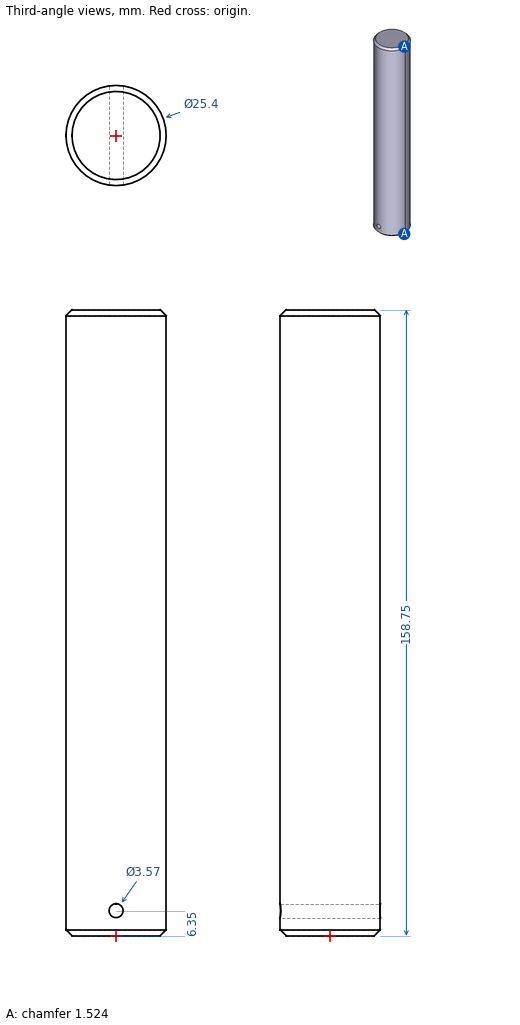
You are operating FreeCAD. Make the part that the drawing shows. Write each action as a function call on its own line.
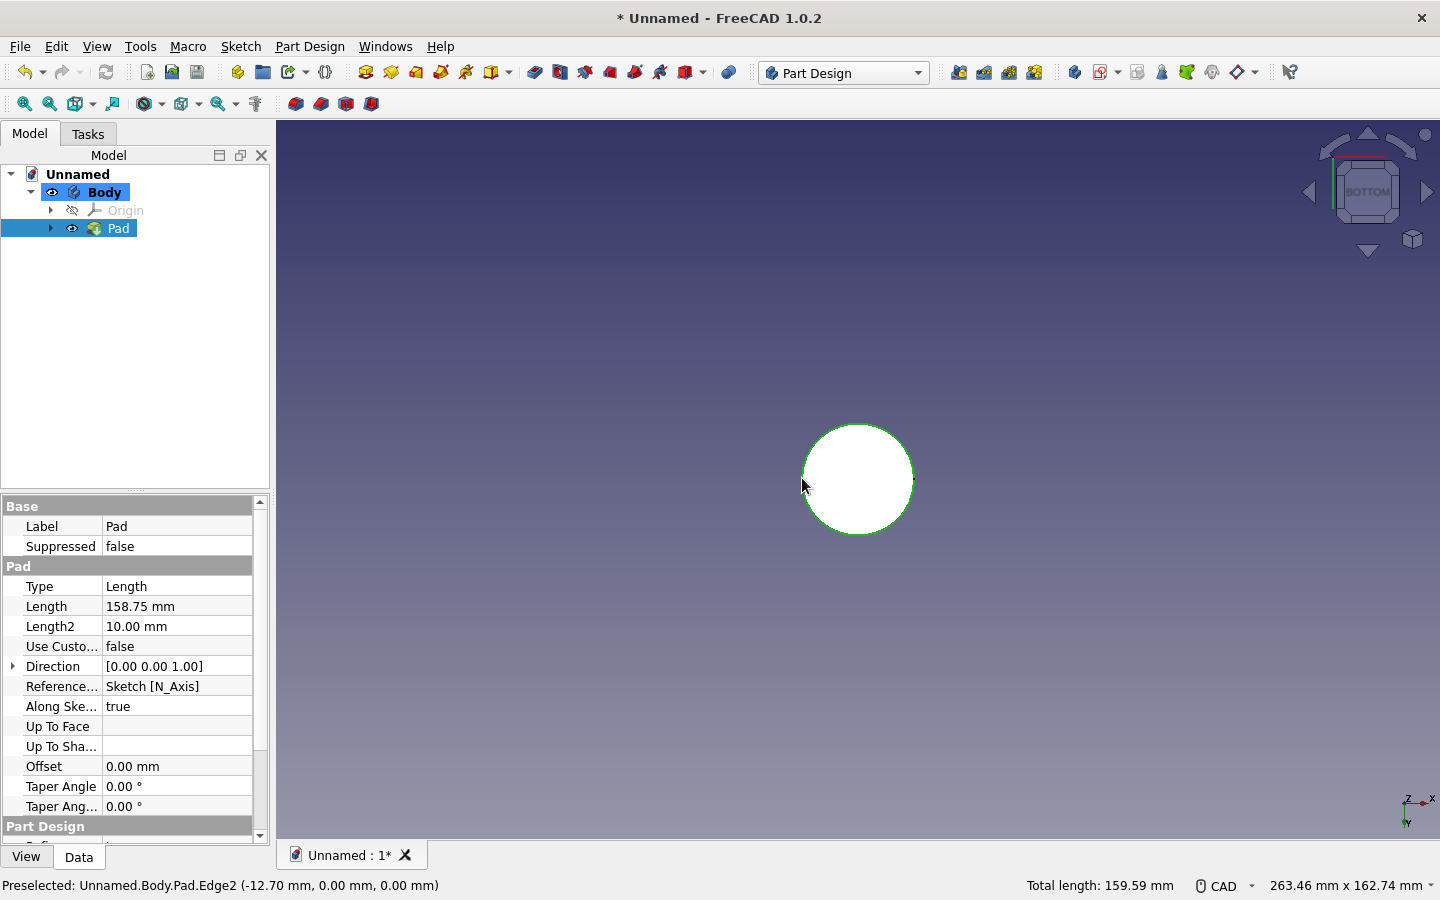
click(321, 104)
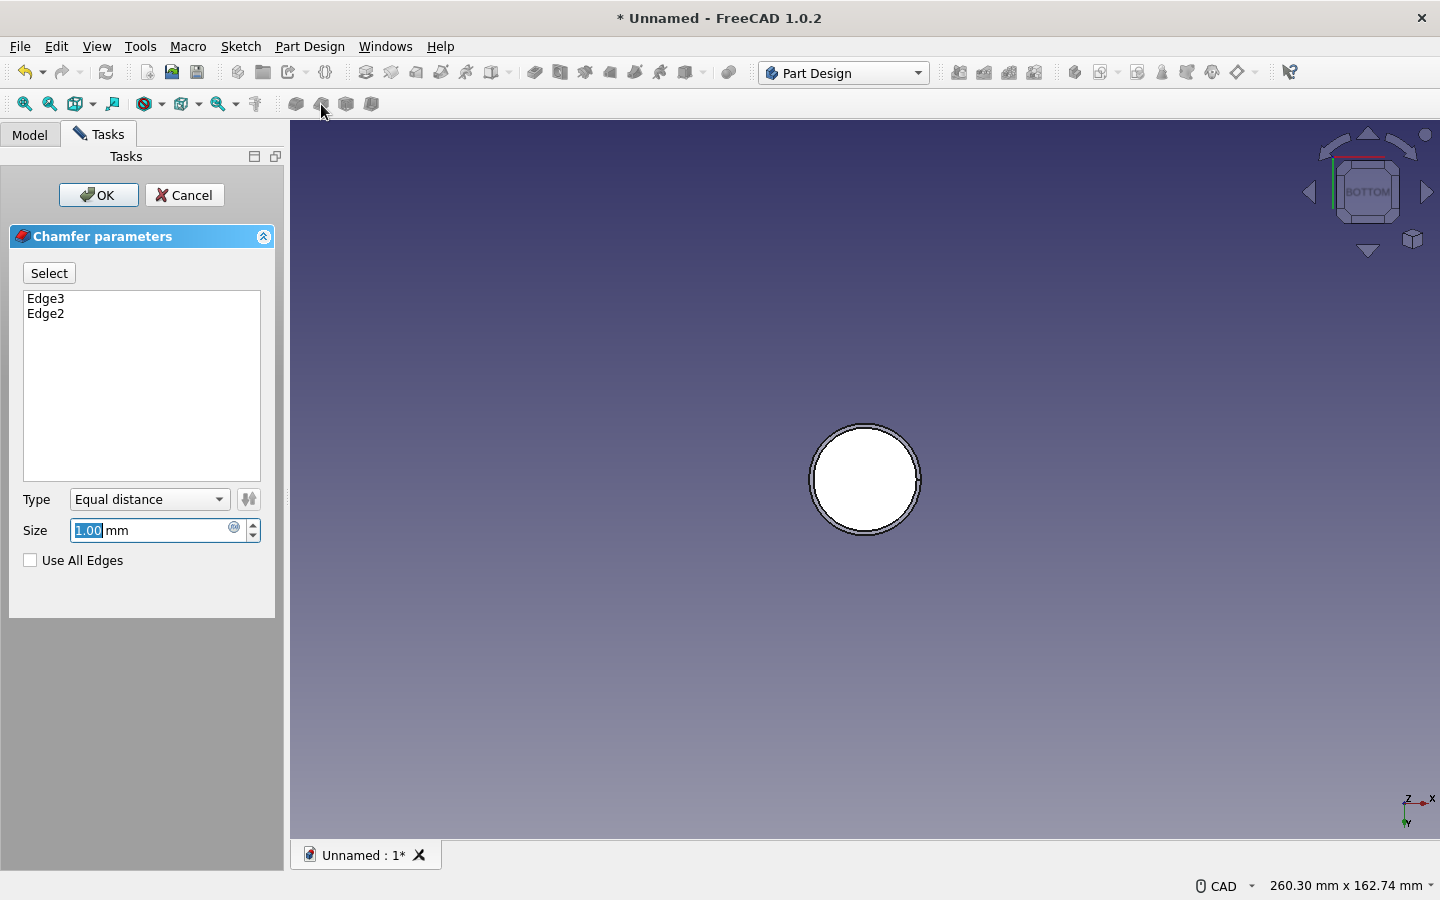
text(1.524)
key(Tab)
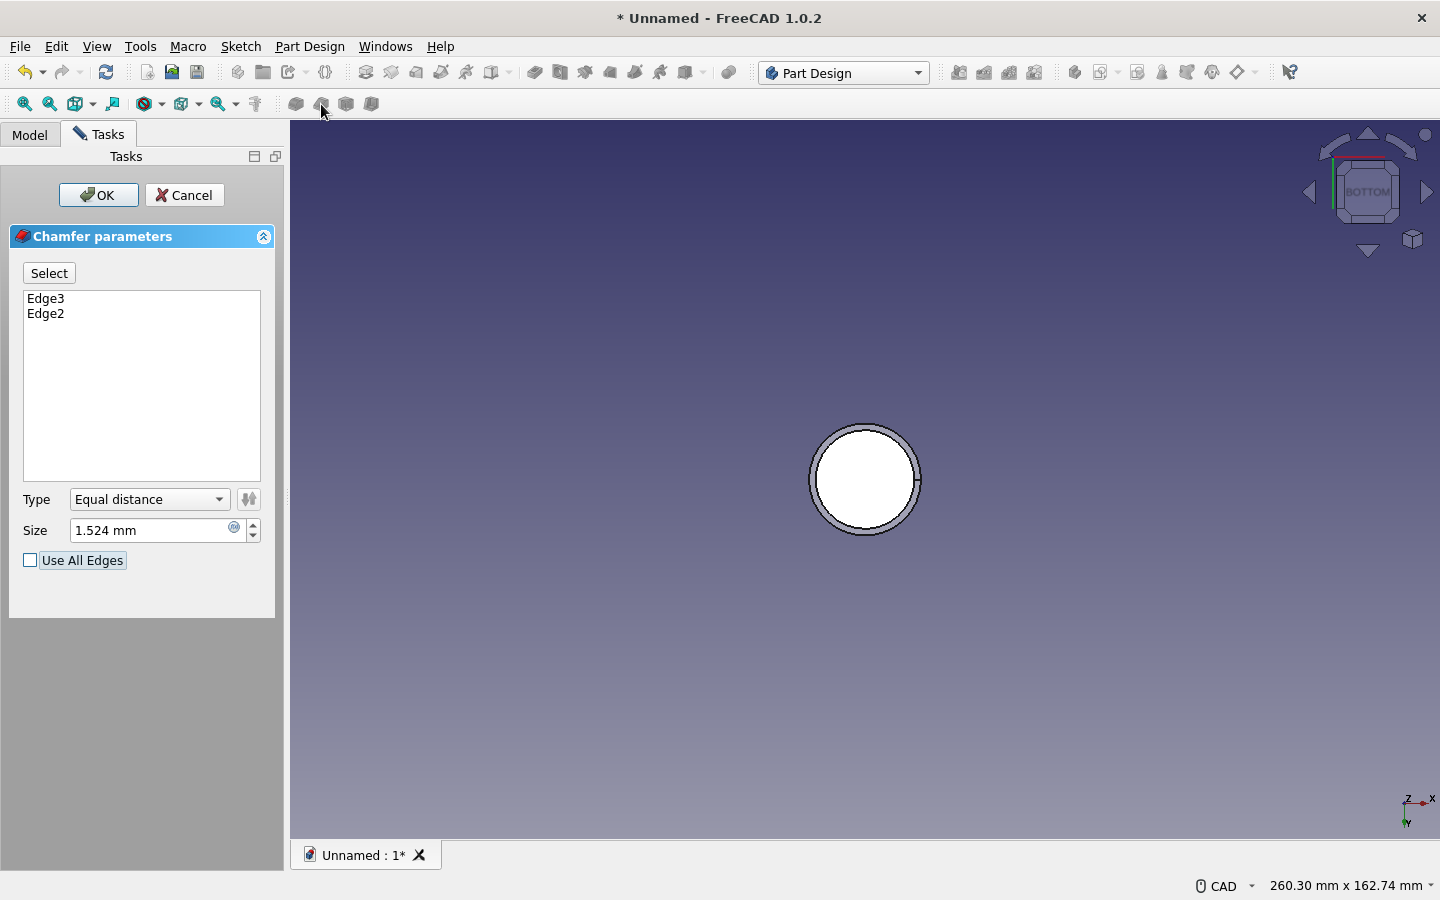
click(99, 195)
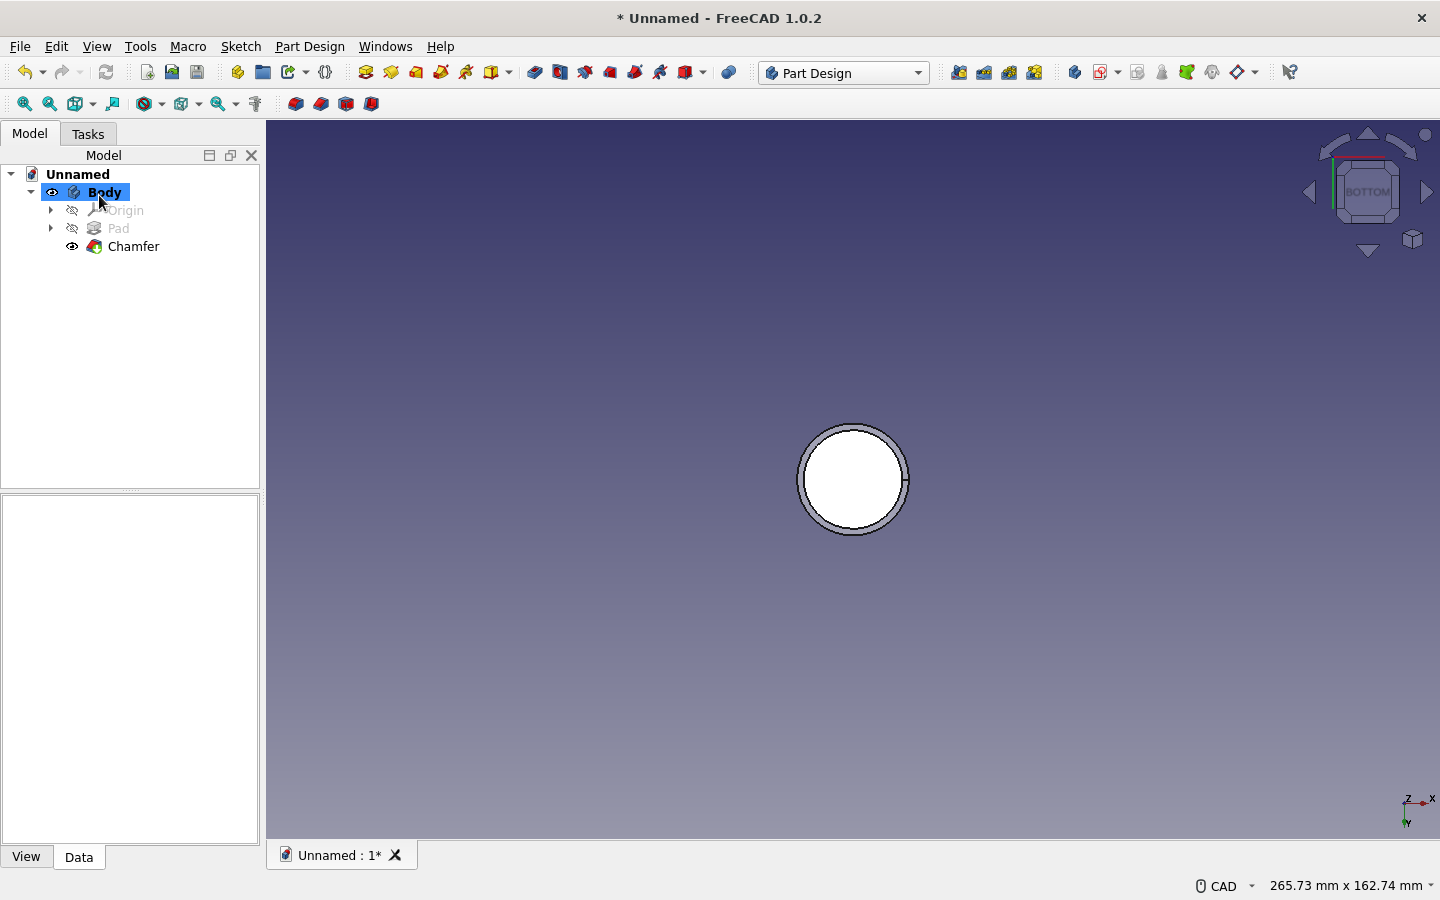
key(v)
key(f)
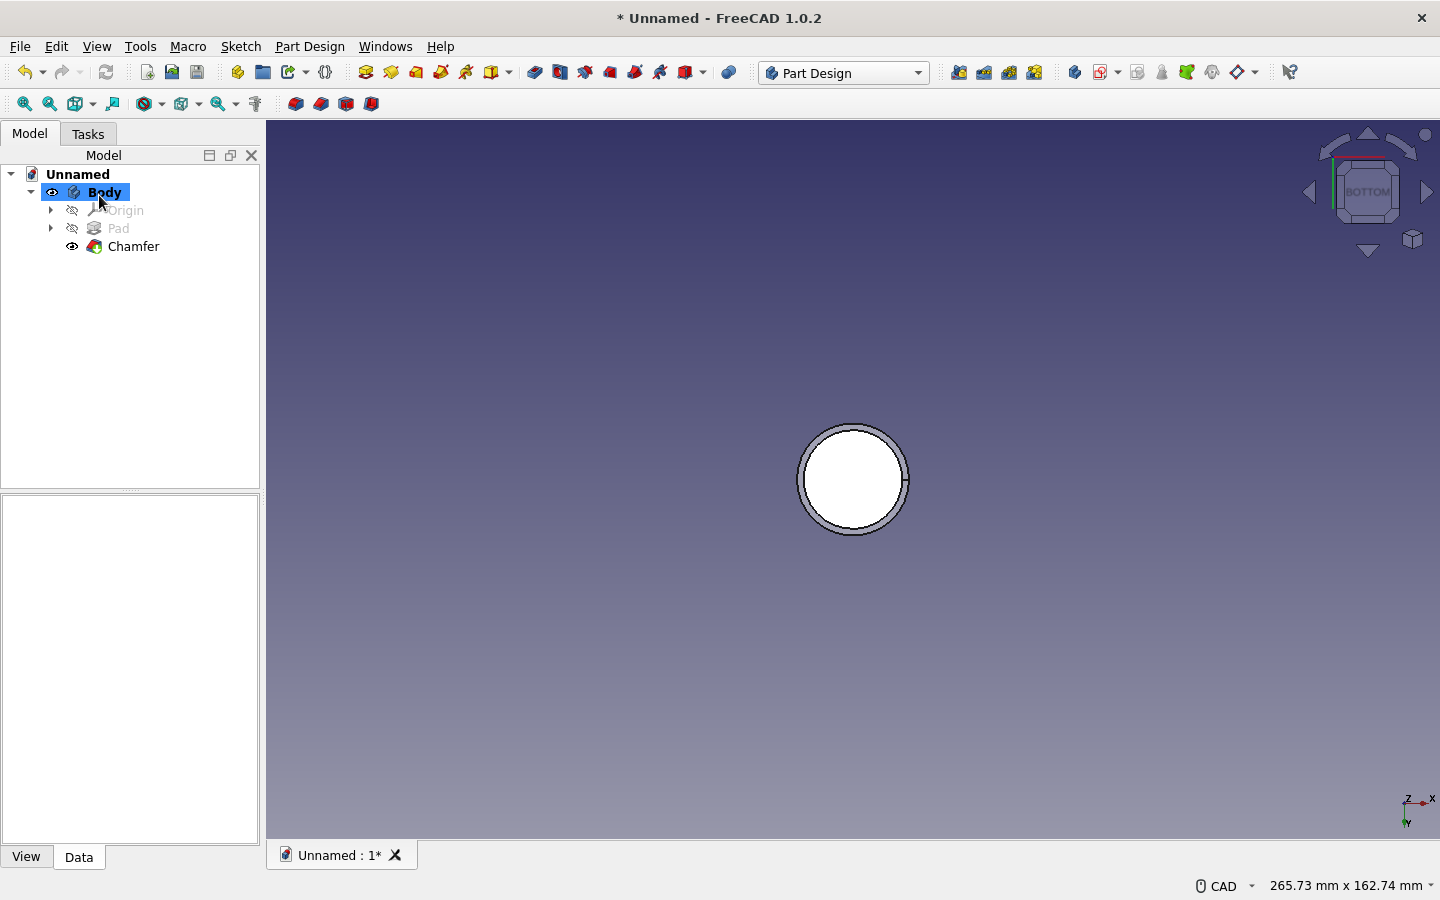
click(1100, 72)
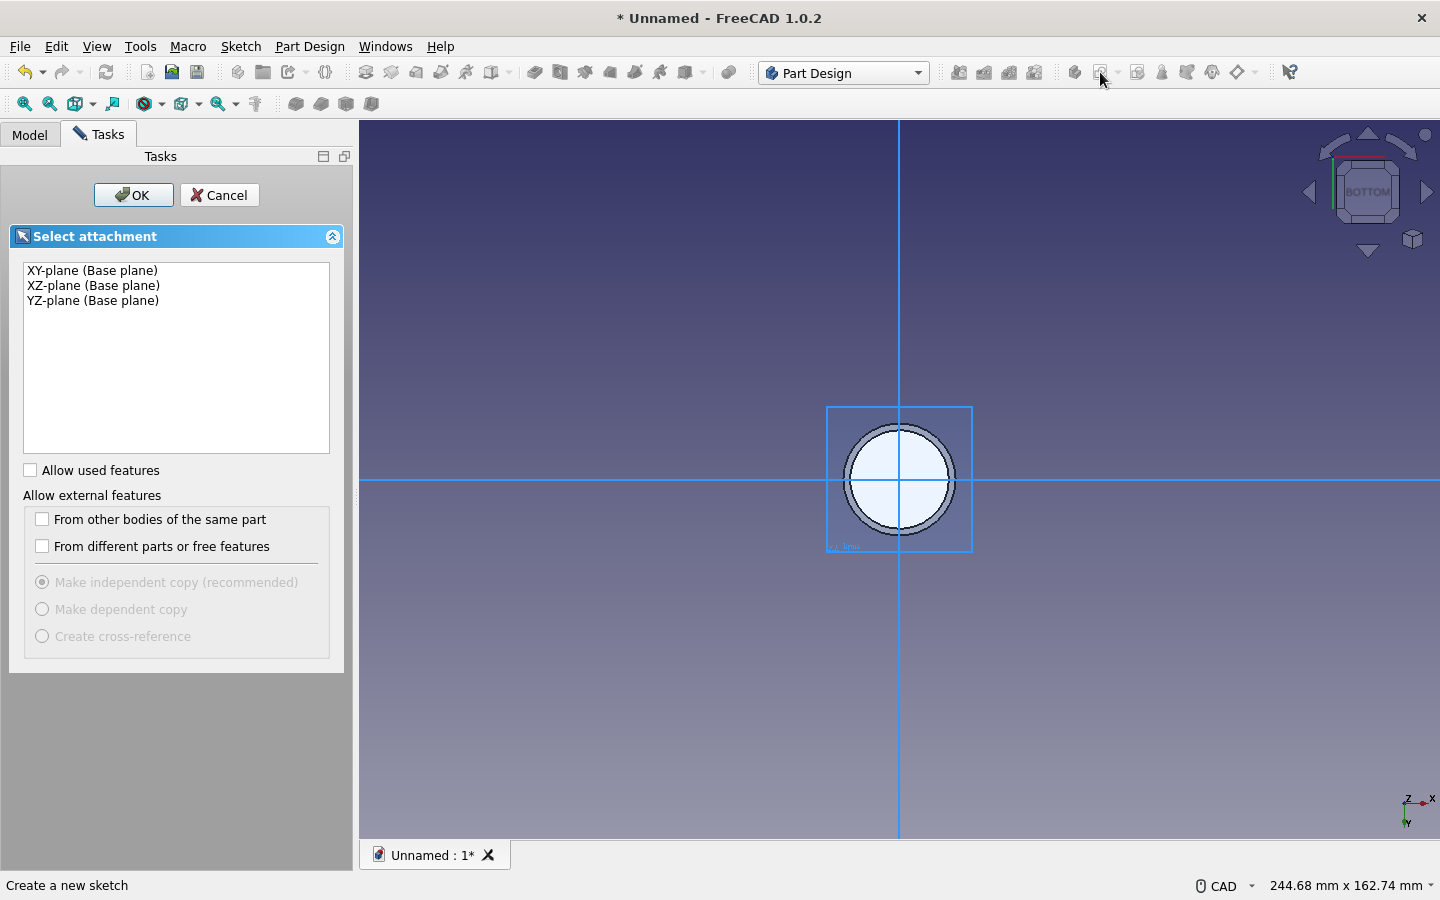
click(84, 286)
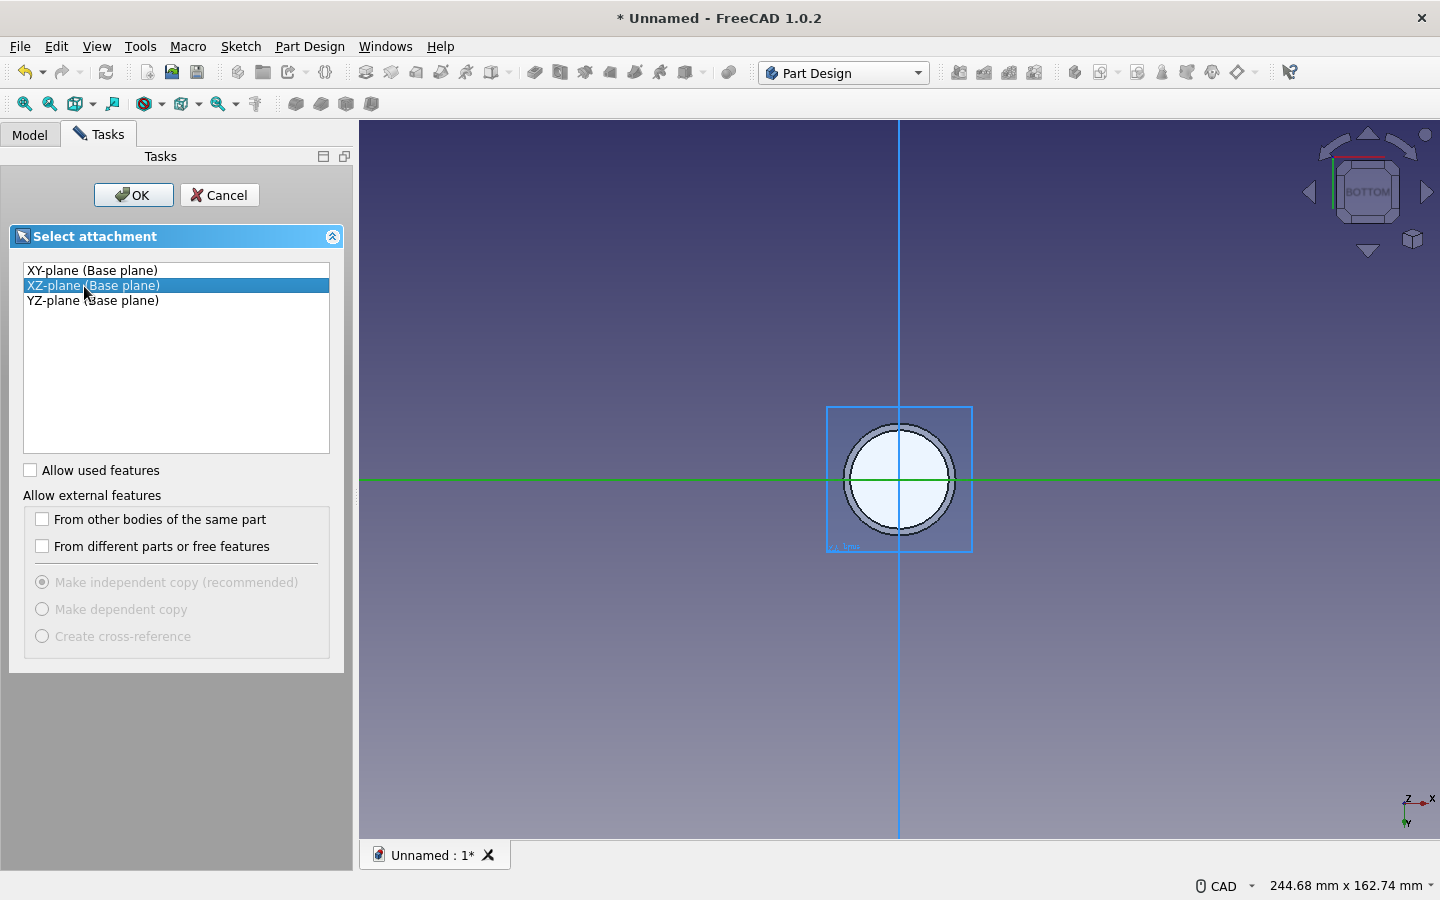
click(134, 195)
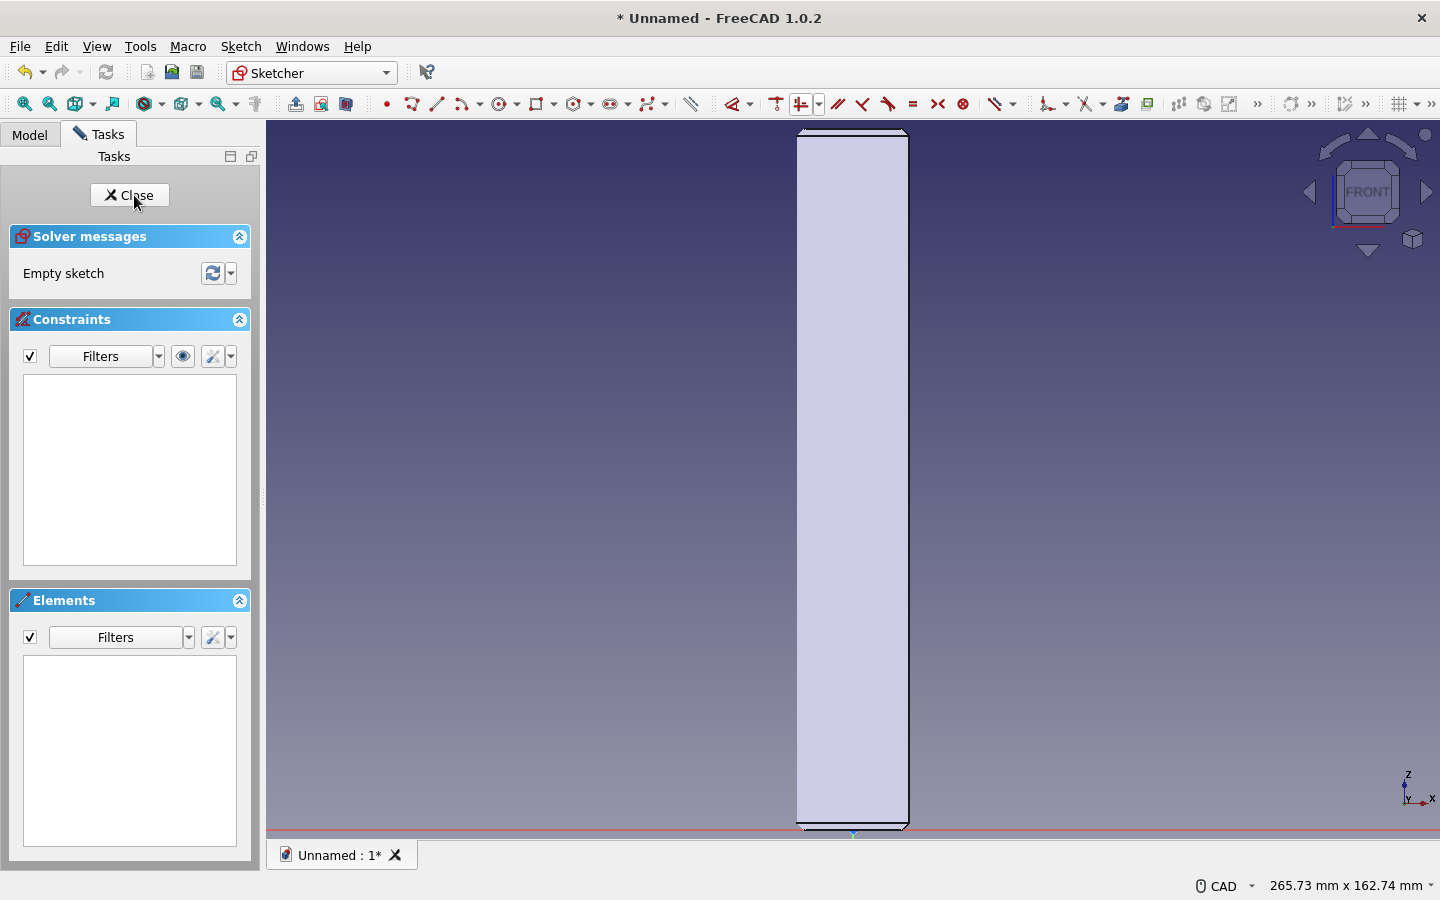
key(q)
key(s)